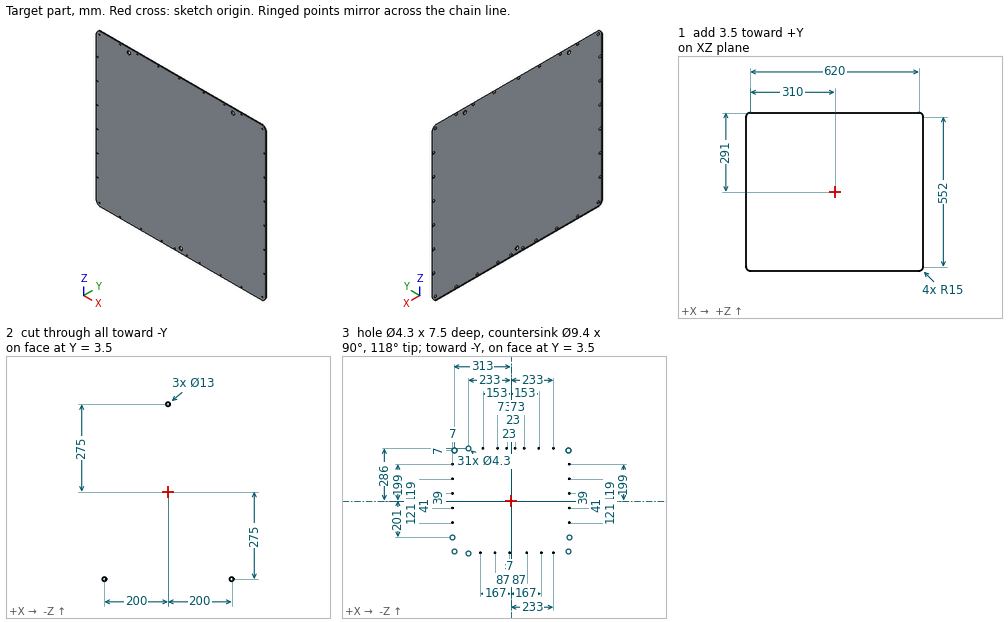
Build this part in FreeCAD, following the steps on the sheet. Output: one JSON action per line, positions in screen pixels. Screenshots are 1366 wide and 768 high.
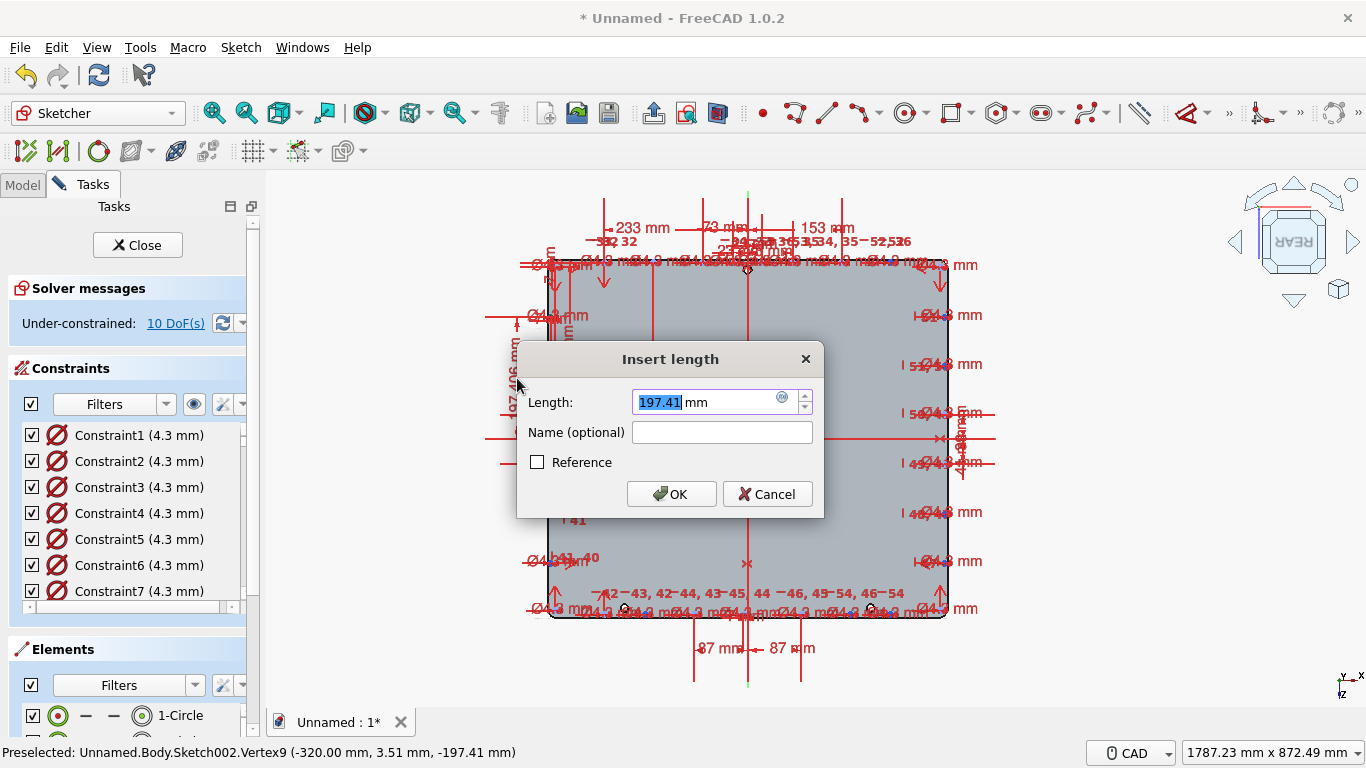
{"action": "type", "text": "199"}
{"action": "key", "text": "Return"}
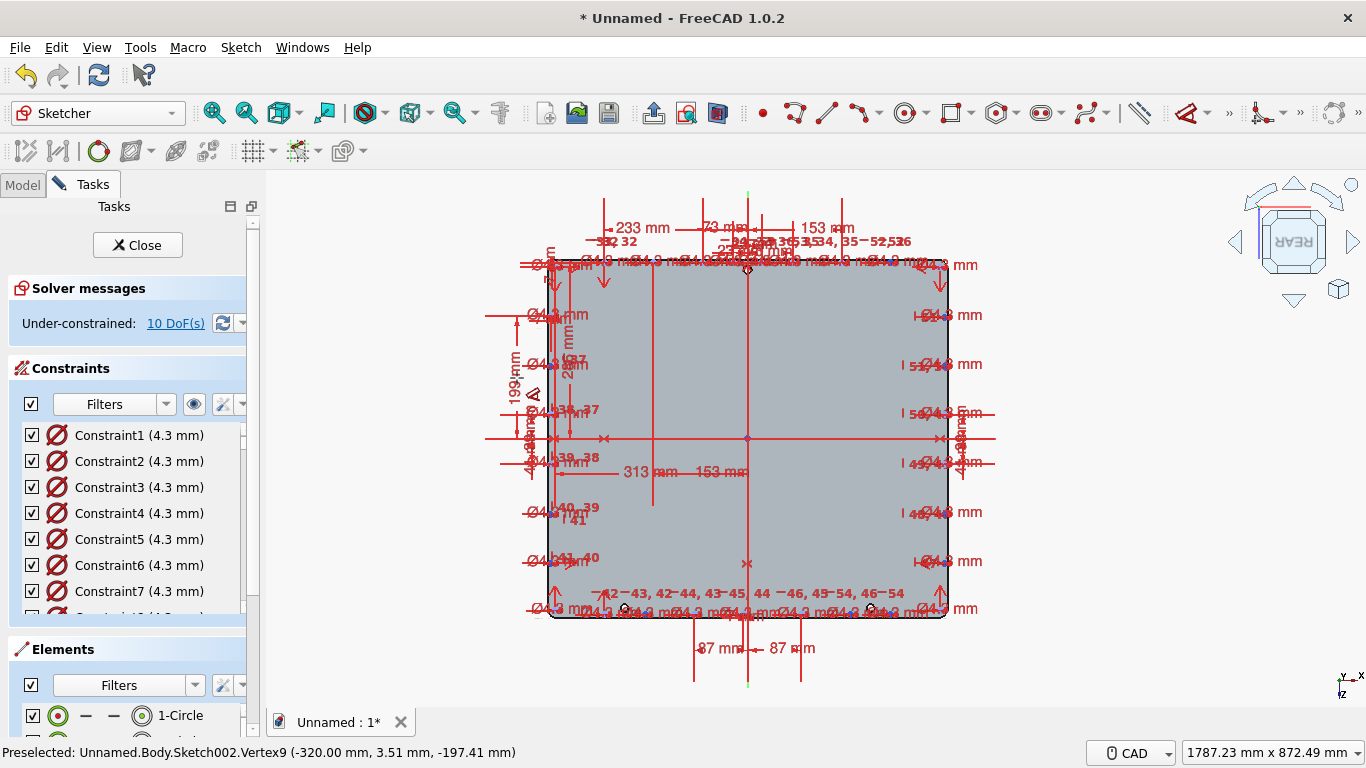
{"action": "left_click", "coordinate": [551, 366]}
{"action": "left_click", "coordinate": [517, 403]}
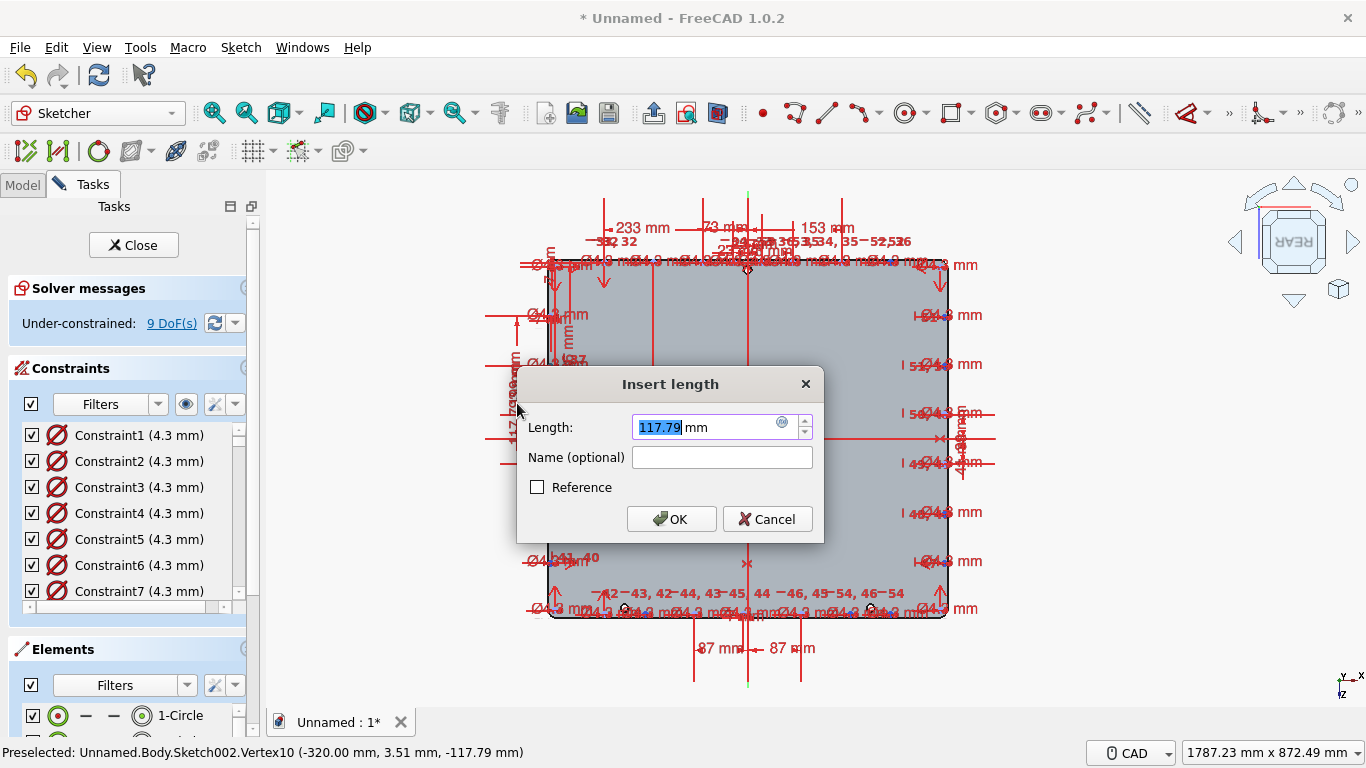
{"action": "type", "text": "119"}
{"action": "key", "text": "Return"}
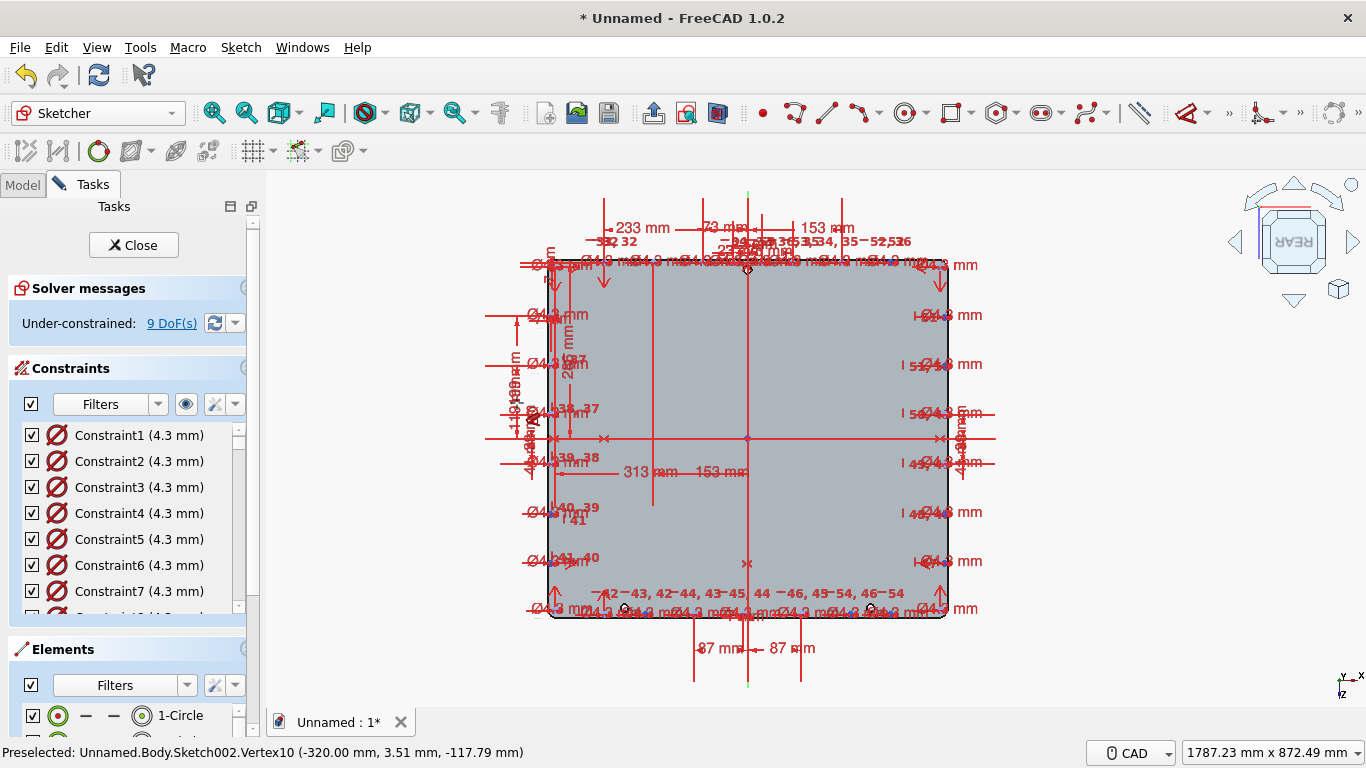
{"action": "left_click", "coordinate": [551, 514]}
{"action": "left_click", "coordinate": [517, 477]}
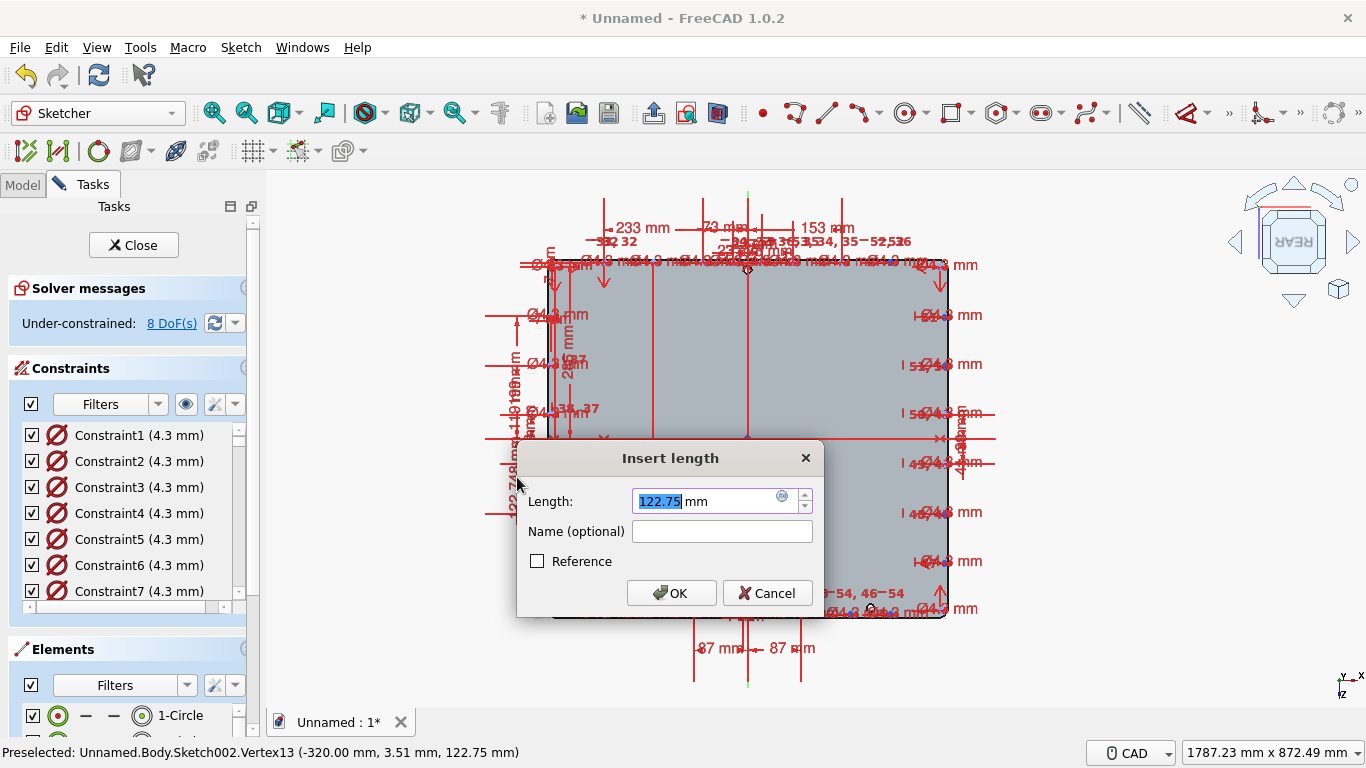
{"action": "type", "text": "121"}
{"action": "key", "text": "Return"}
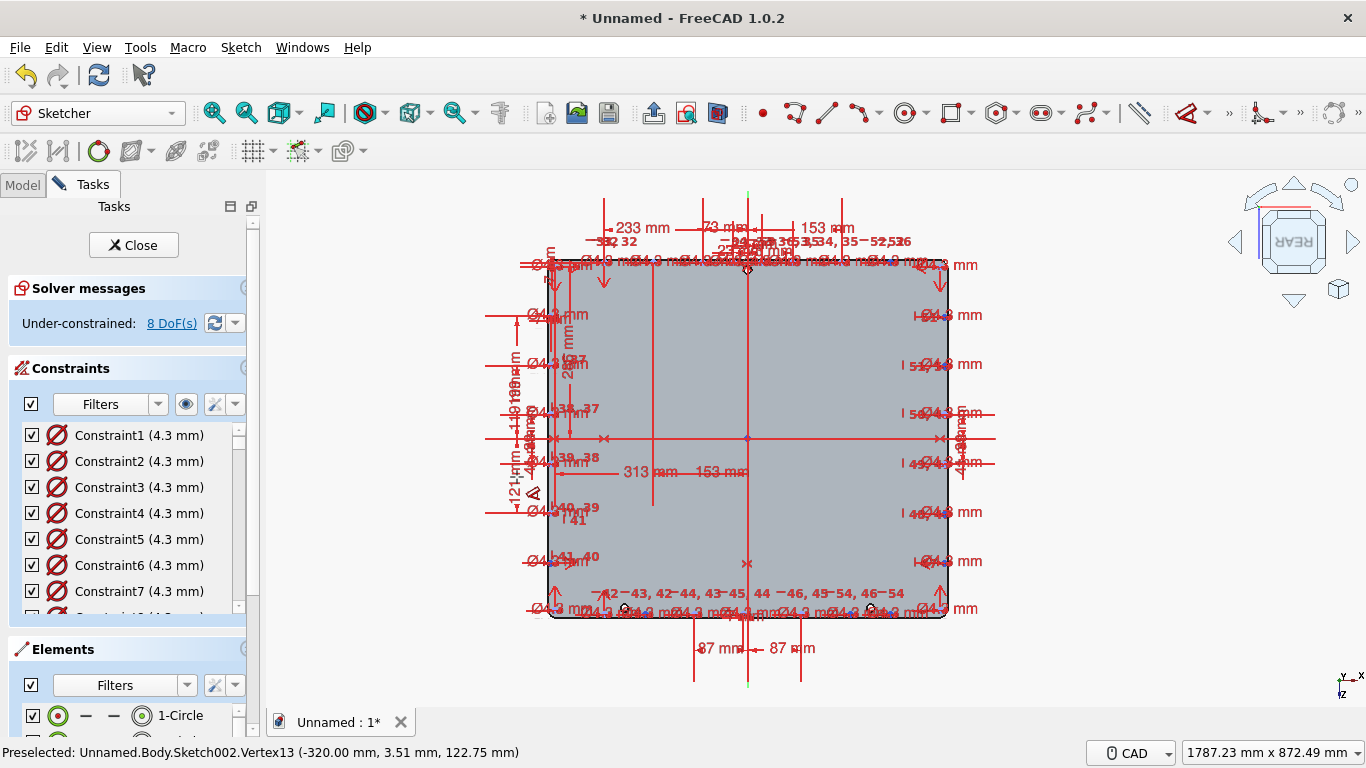
{"action": "left_click", "coordinate": [551, 563]}
{"action": "left_click", "coordinate": [517, 501]}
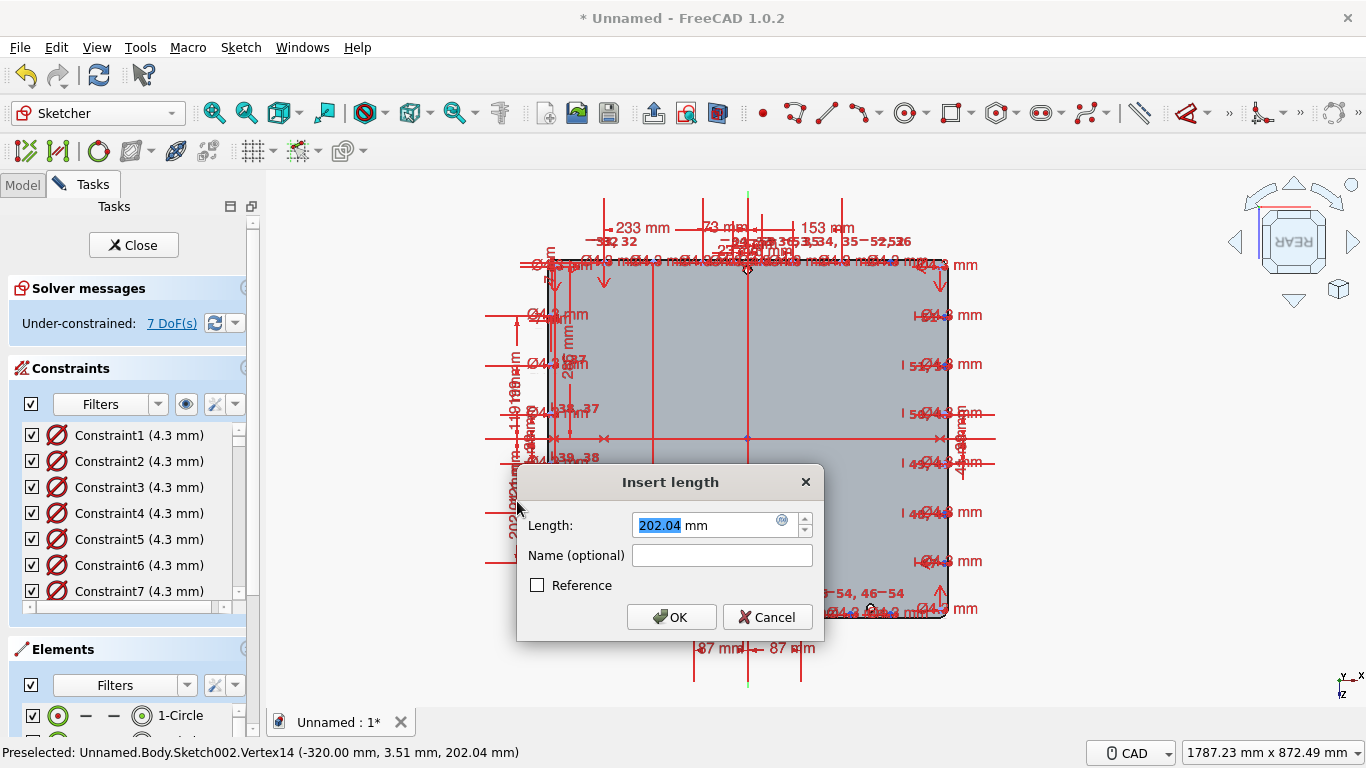
{"action": "type", "text": "201"}
{"action": "key", "text": "Return"}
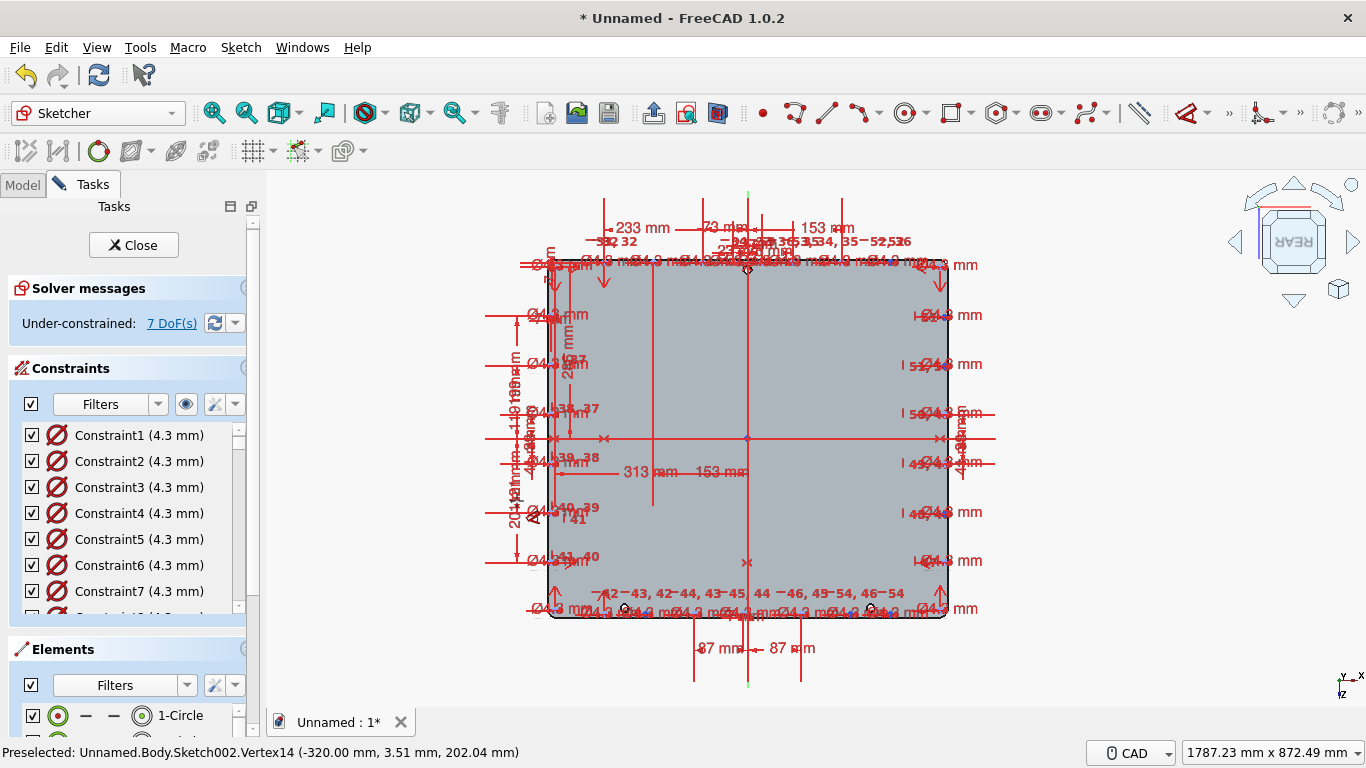
{"action": "left_click", "coordinate": [645, 615]}
{"action": "left_click", "coordinate": [696, 405]}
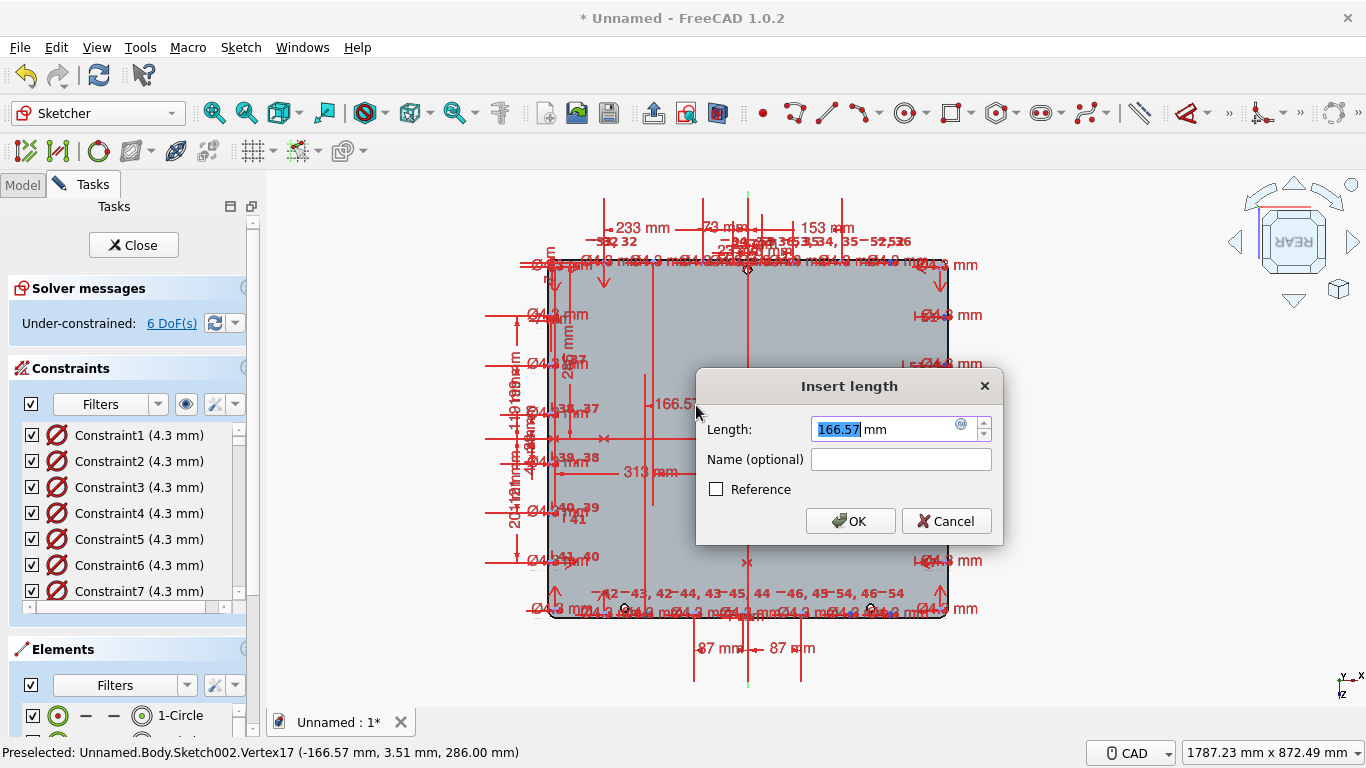
{"action": "type", "text": "167"}
{"action": "key", "text": "Return"}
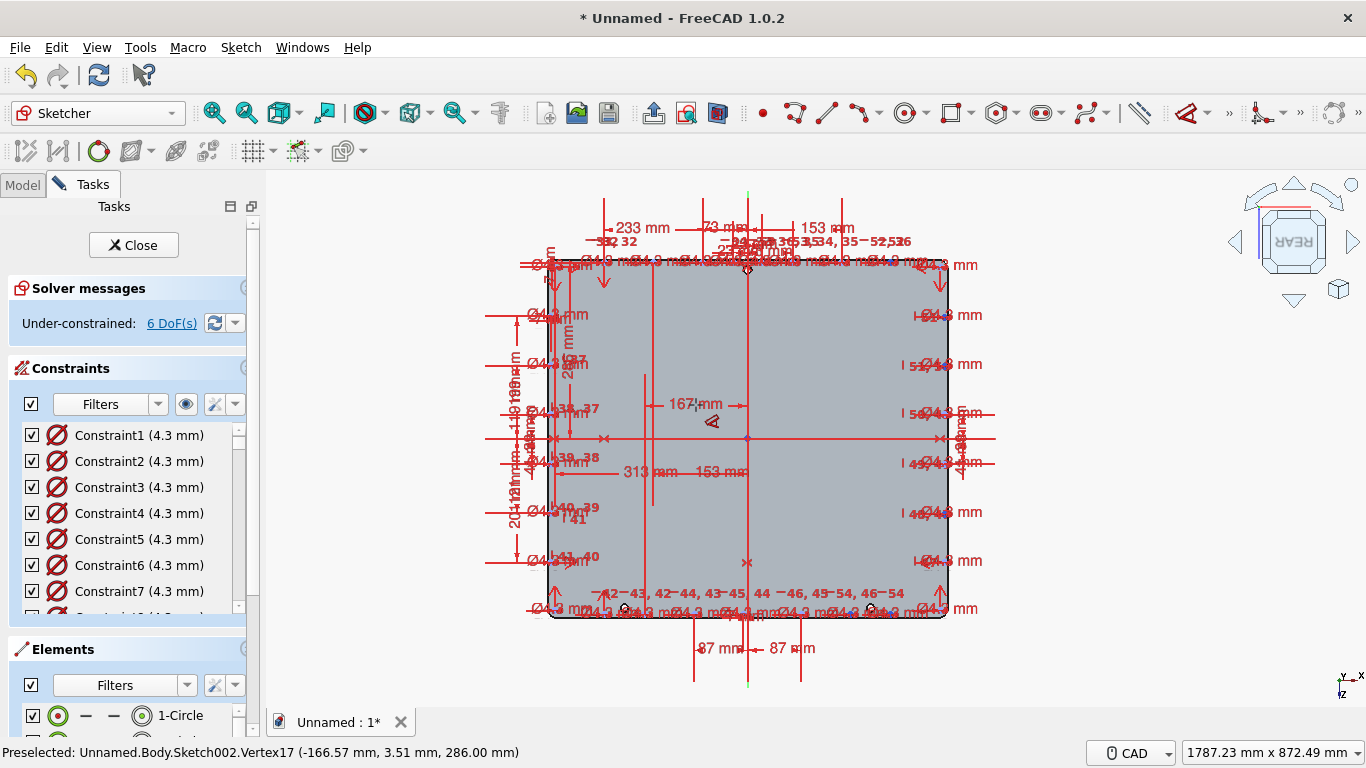
{"action": "left_click", "coordinate": [851, 615]}
{"action": "left_click", "coordinate": [799, 405]}